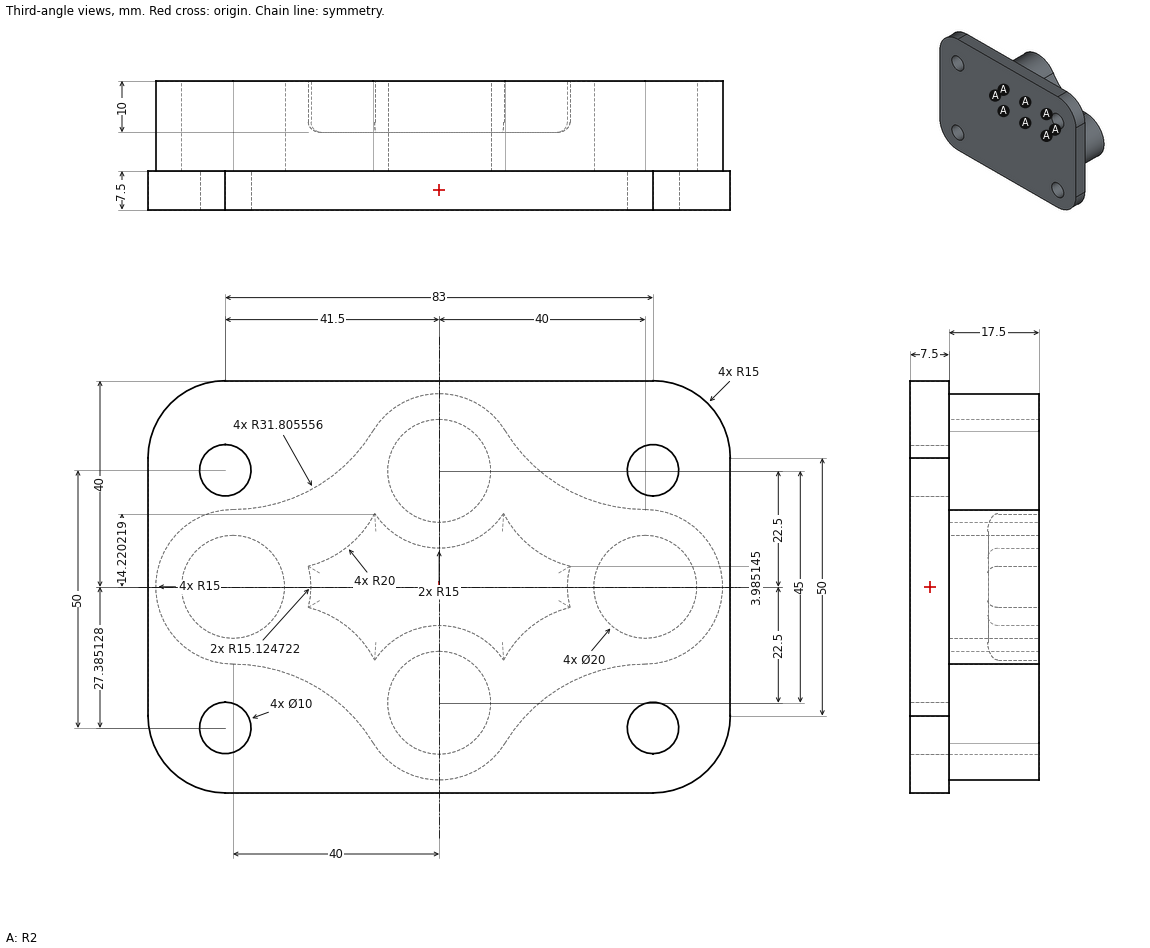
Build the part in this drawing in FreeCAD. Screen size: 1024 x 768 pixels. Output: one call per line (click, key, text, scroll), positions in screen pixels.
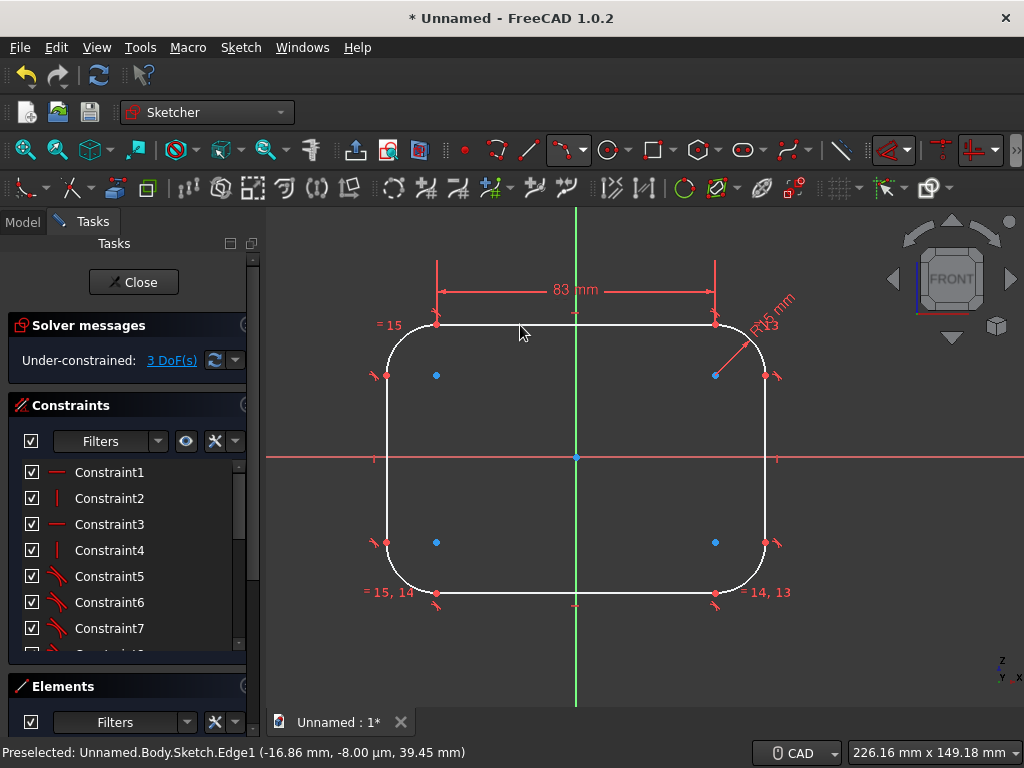
click(765, 425)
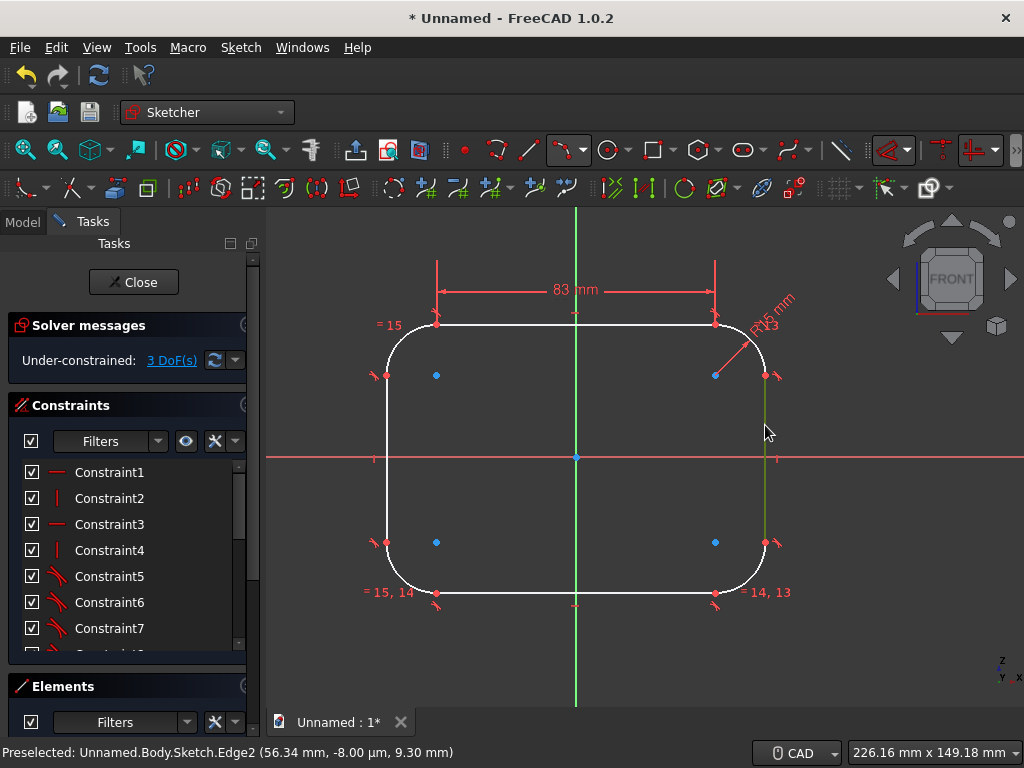
key(i)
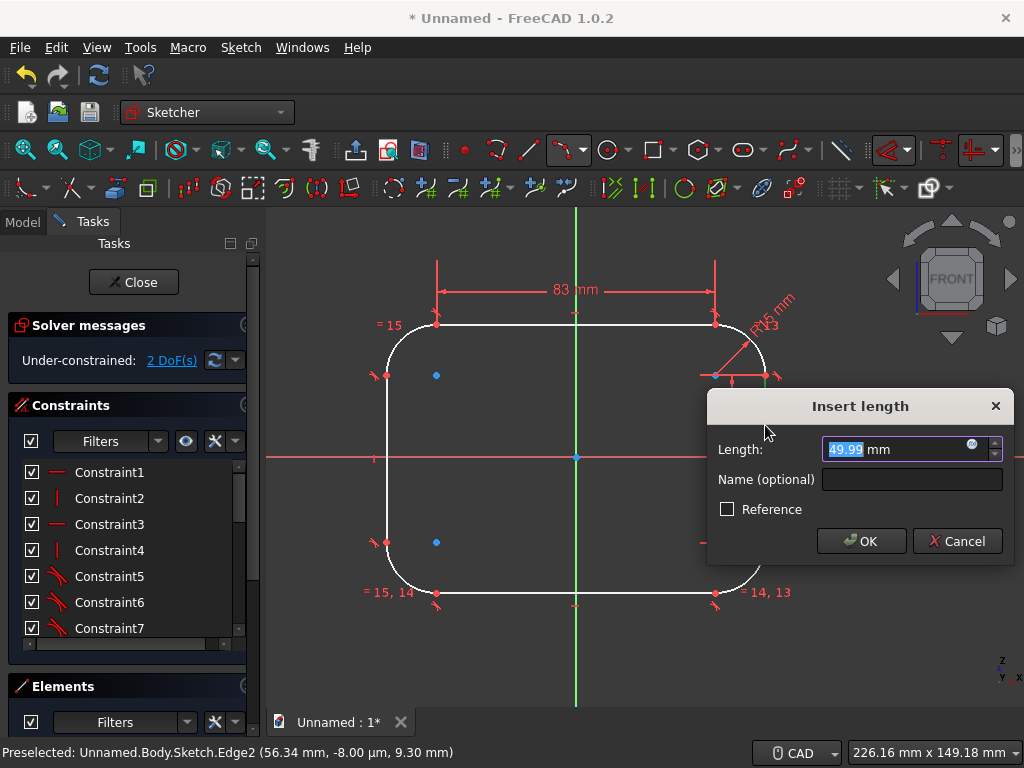
text(50)
key(Return)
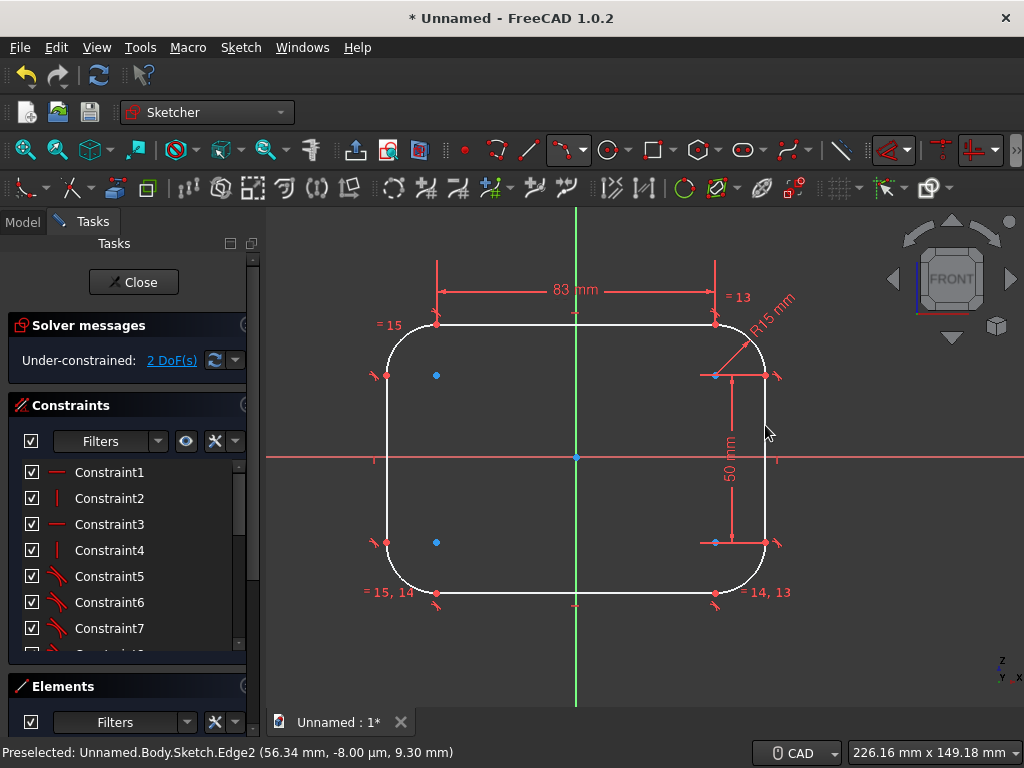
click(437, 325)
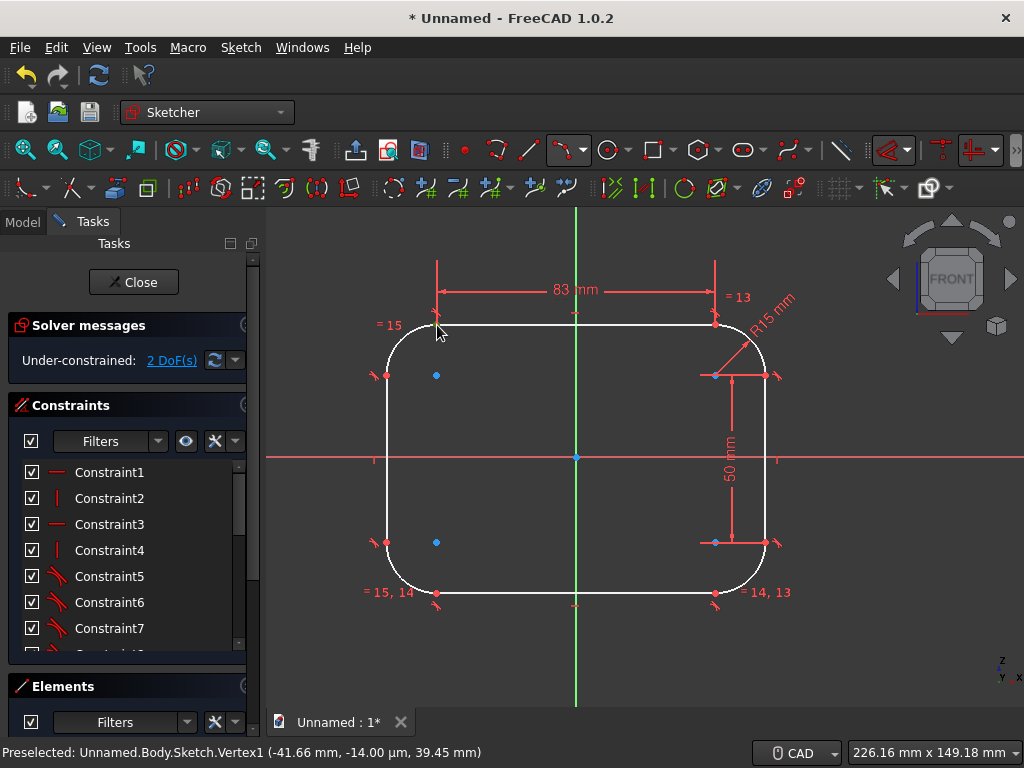
key(i)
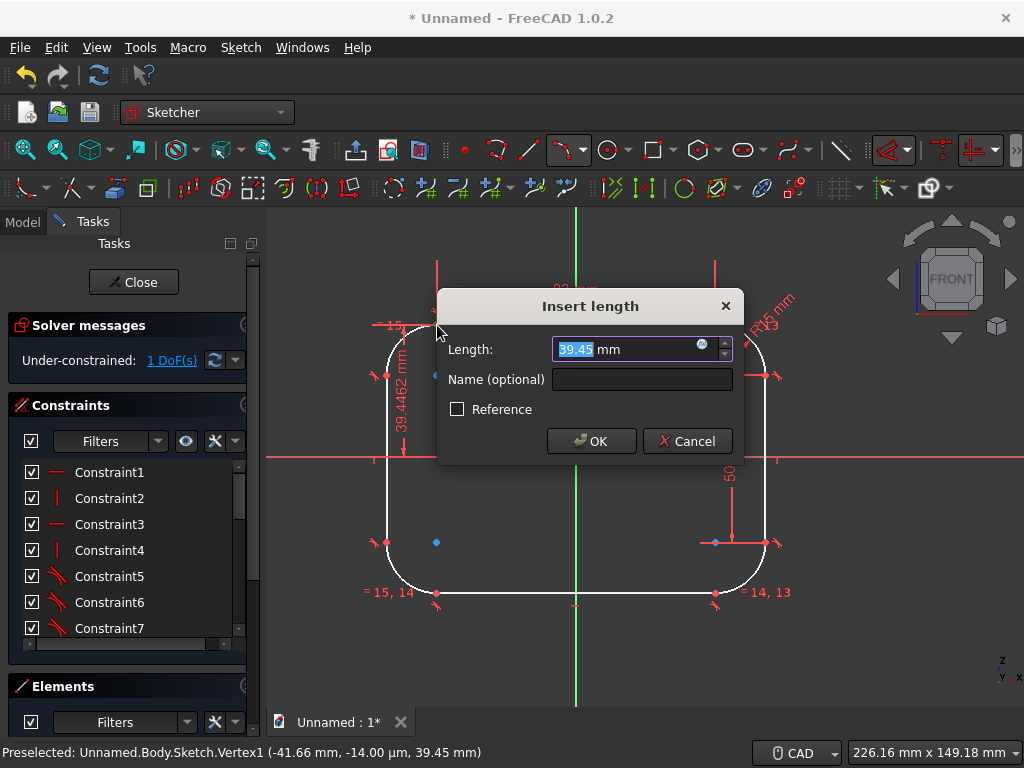
text(40)
key(Return)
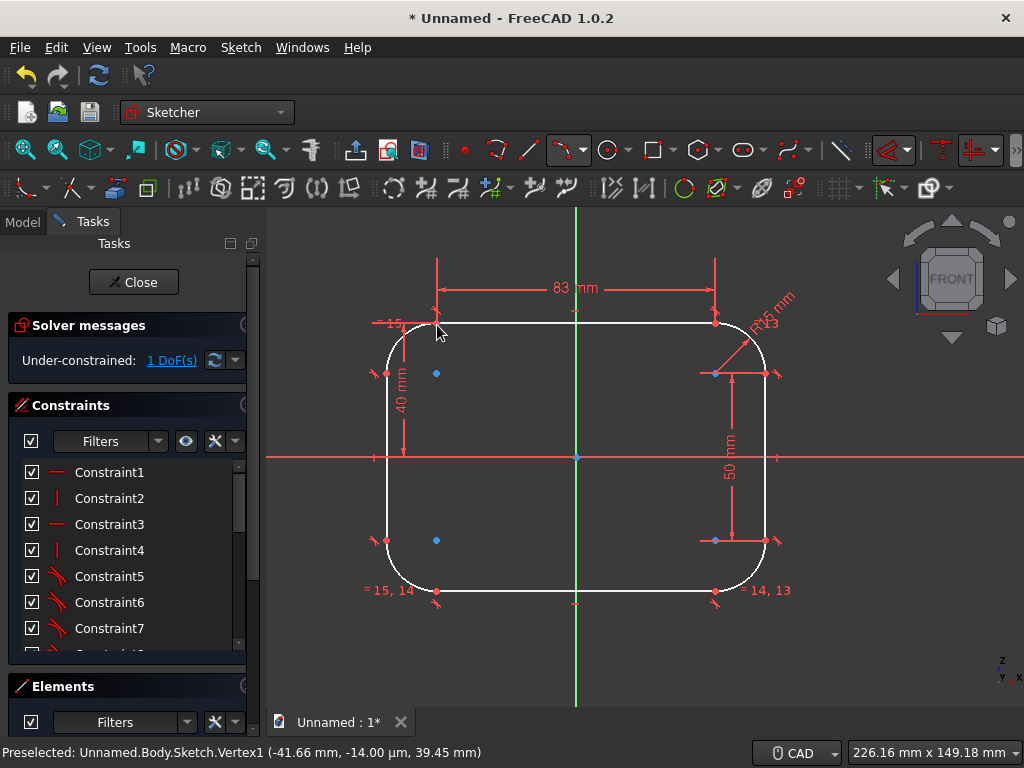
click(437, 323)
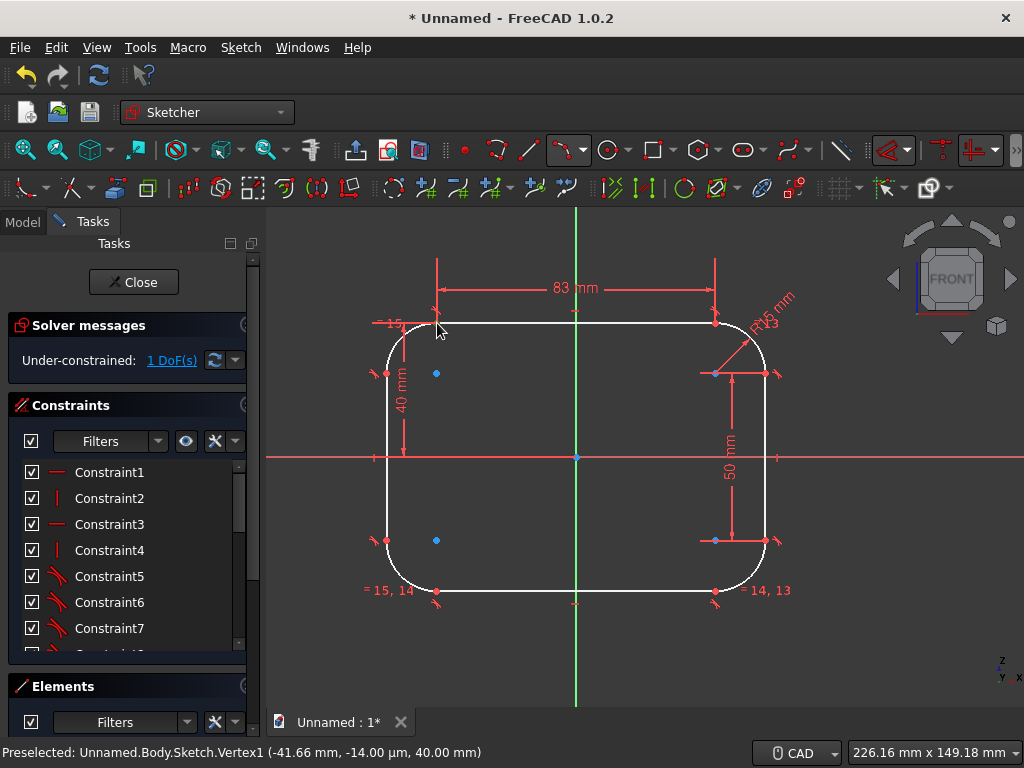
key(l)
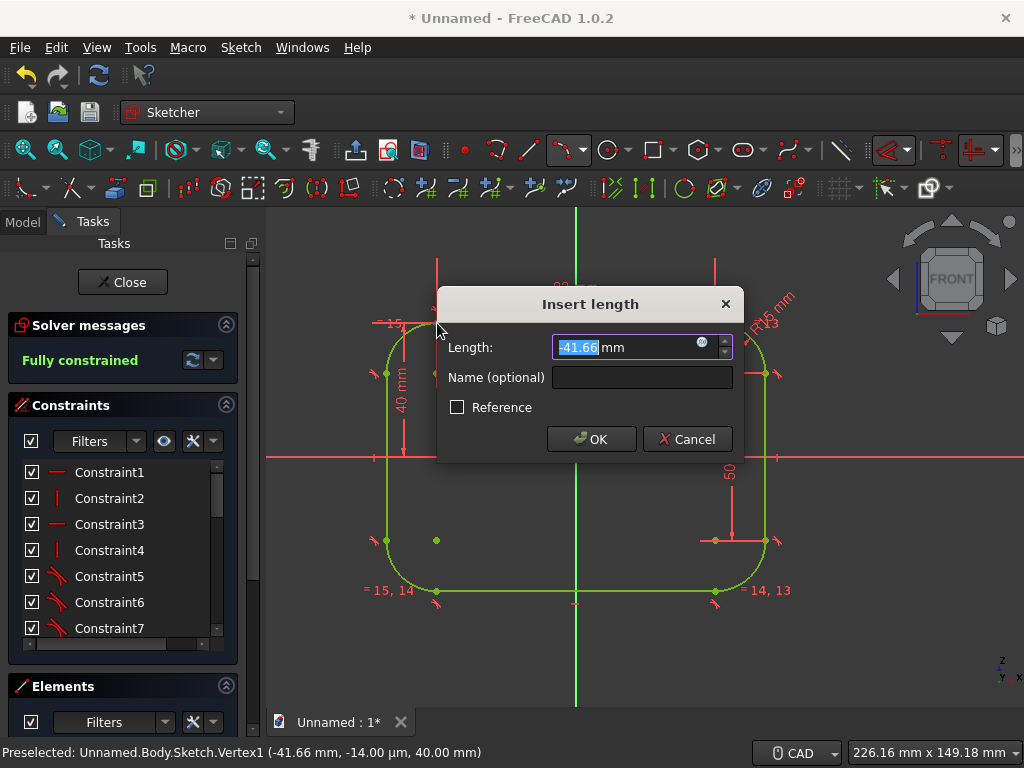
text(-41.5)
key(Return)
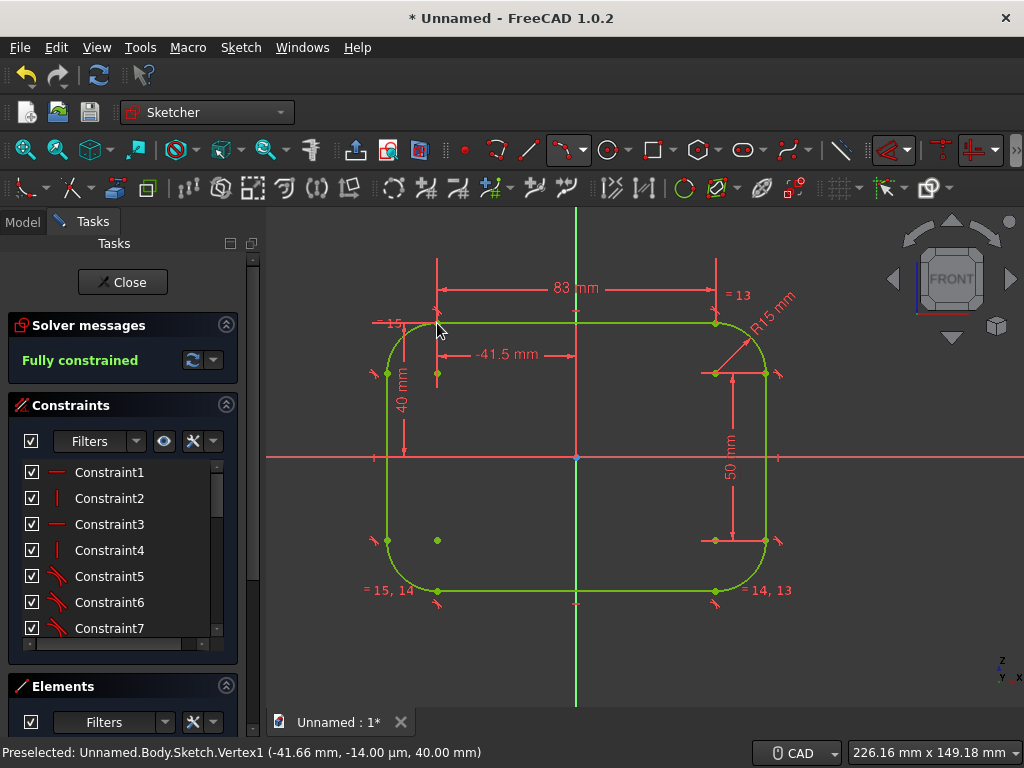
click(123, 282)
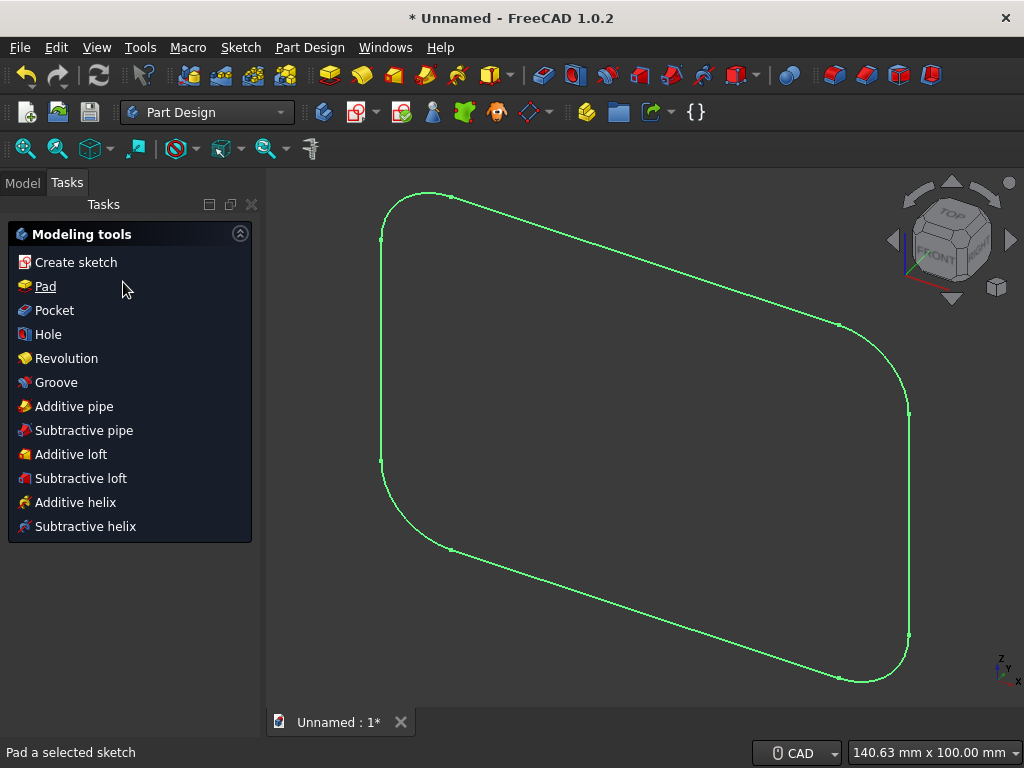
click(330, 76)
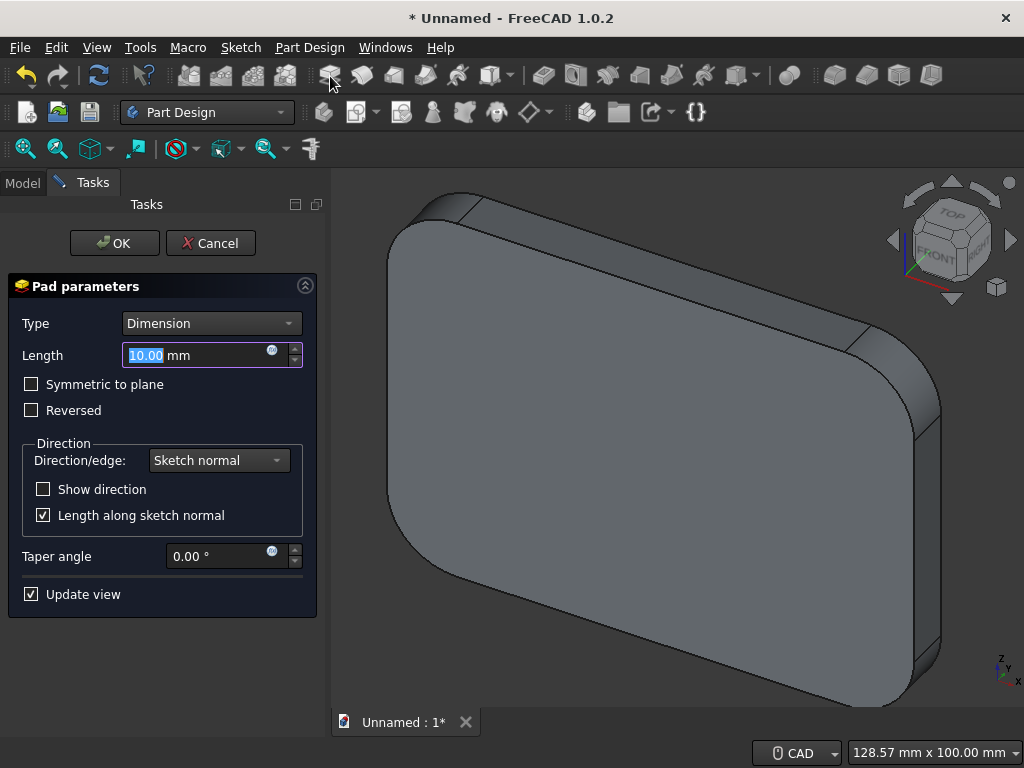
text(7.5)
key(Tab)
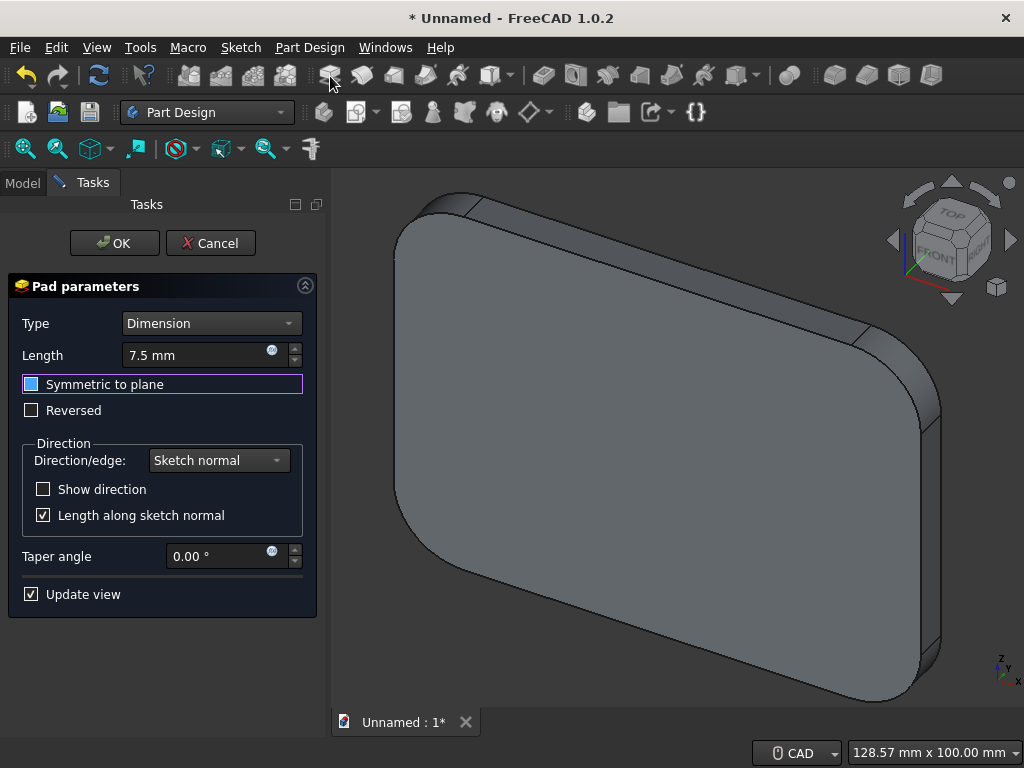
click(30, 384)